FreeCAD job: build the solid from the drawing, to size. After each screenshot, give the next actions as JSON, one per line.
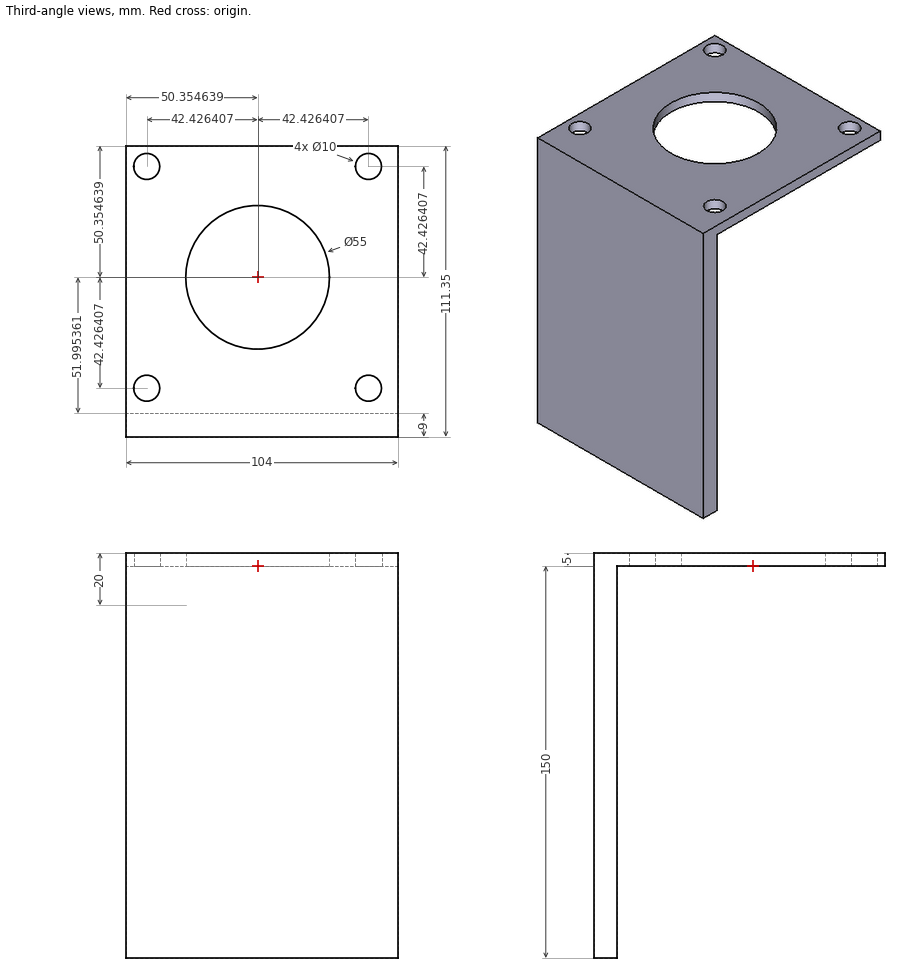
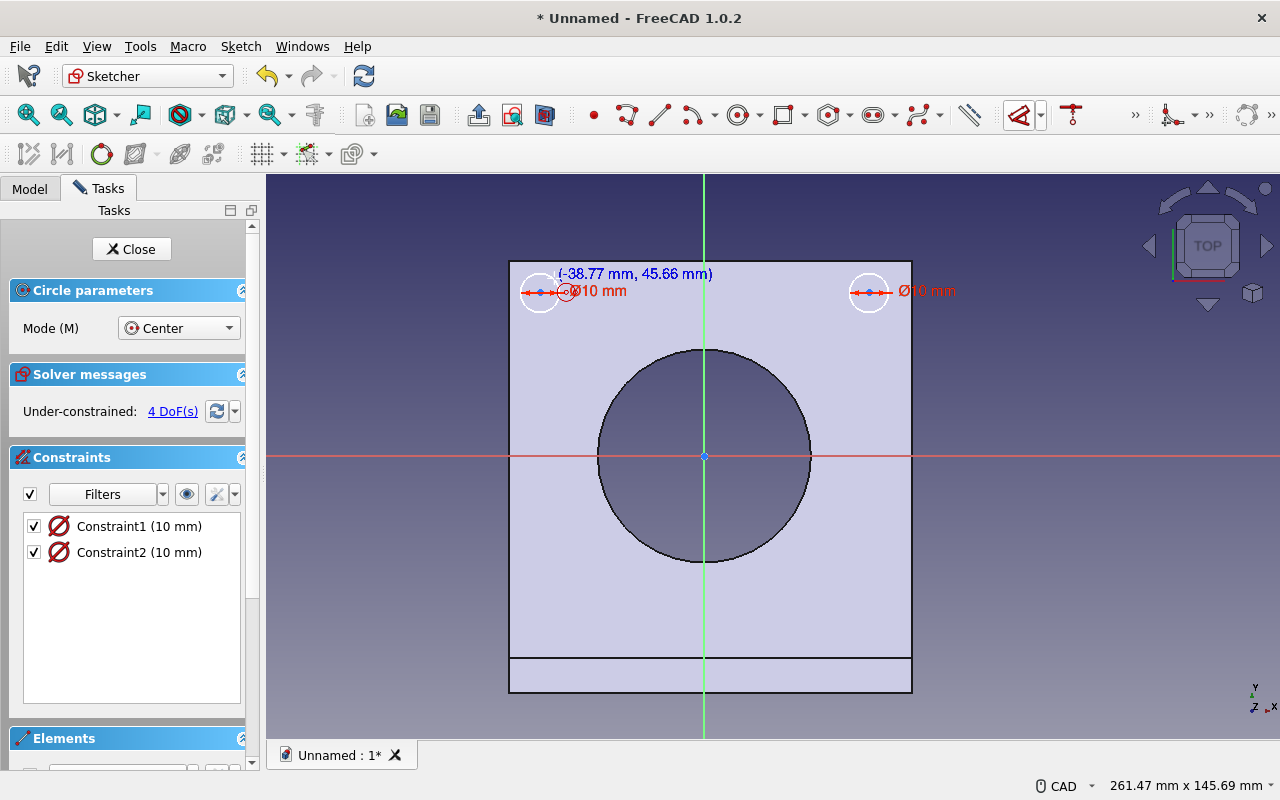
{"action": "left_click", "coordinate": [540, 621]}
{"action": "mouse_move", "coordinate": [554, 607]}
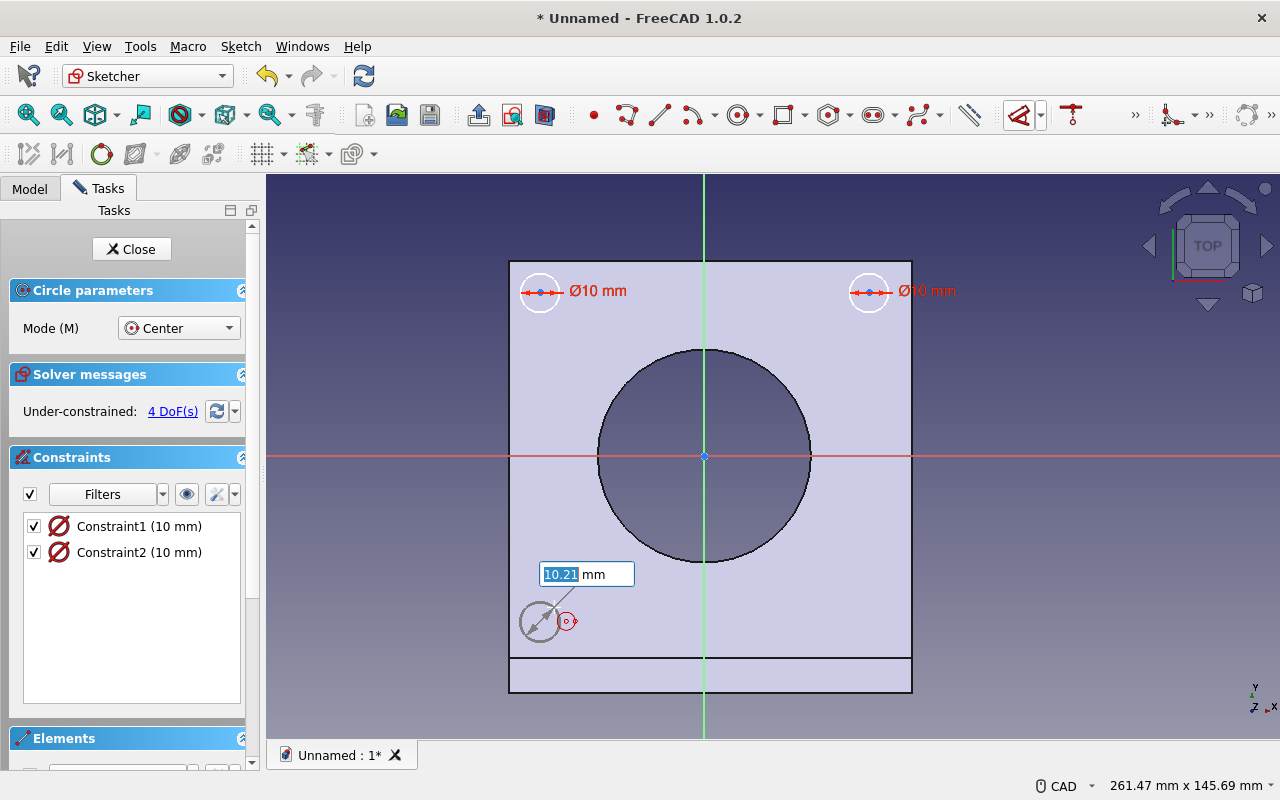
{"action": "type", "text": "10"}
{"action": "key", "text": "Return"}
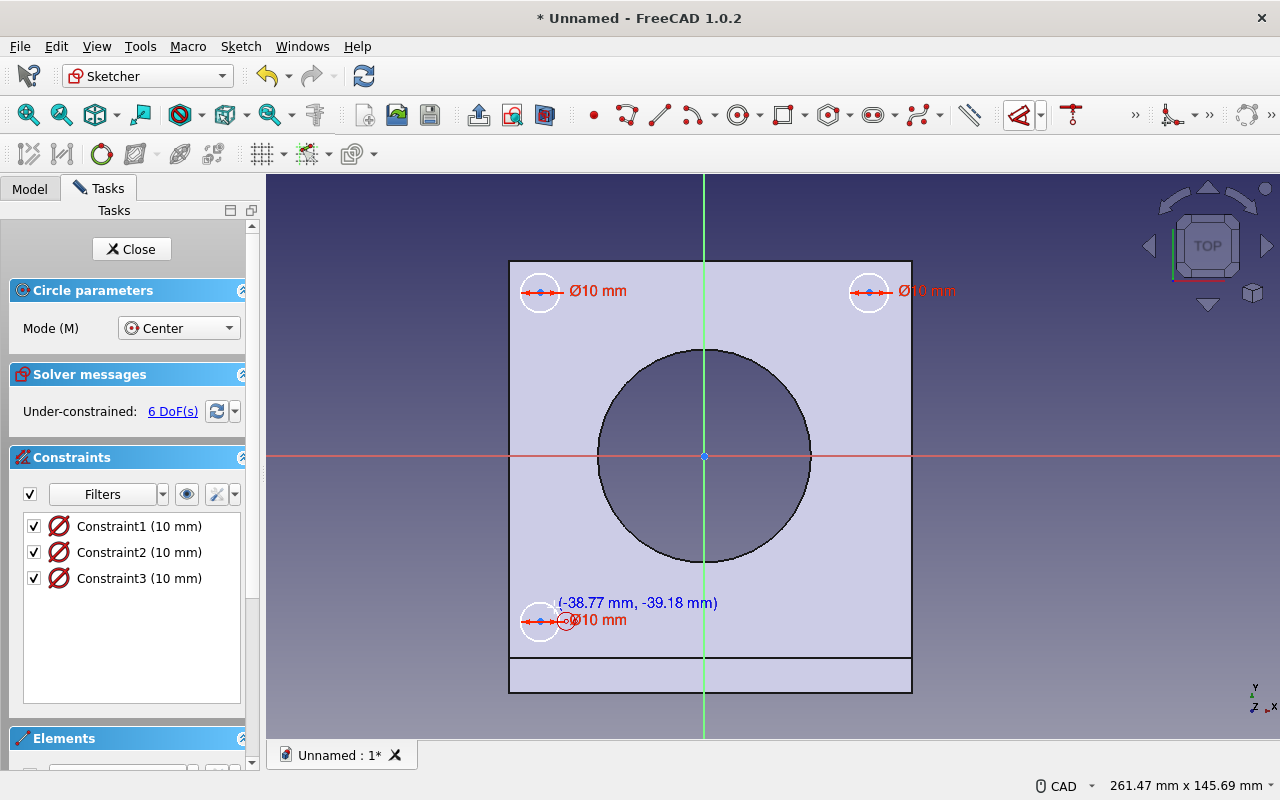
{"action": "left_click", "coordinate": [869, 621]}
{"action": "mouse_move", "coordinate": [883, 607]}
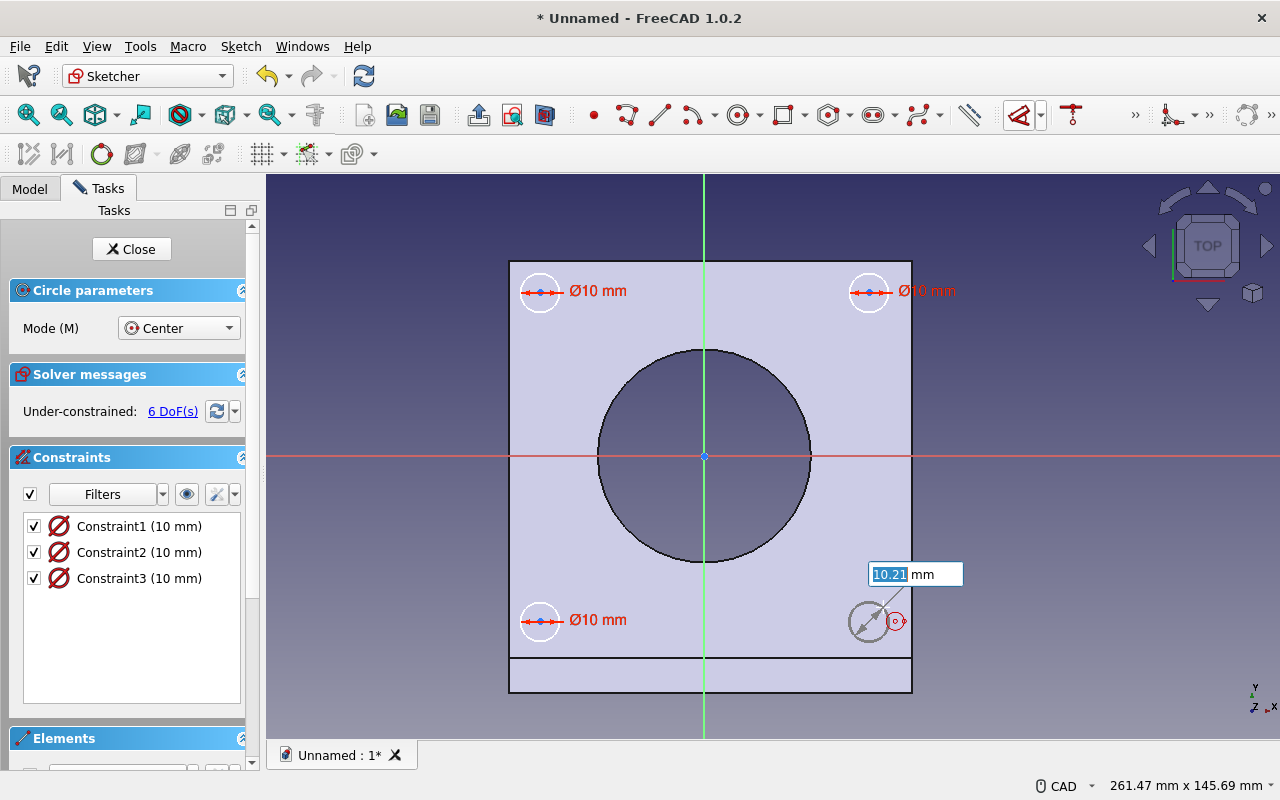
{"action": "type", "text": "10"}
{"action": "key", "text": "Return"}
{"action": "key", "text": "Escape"}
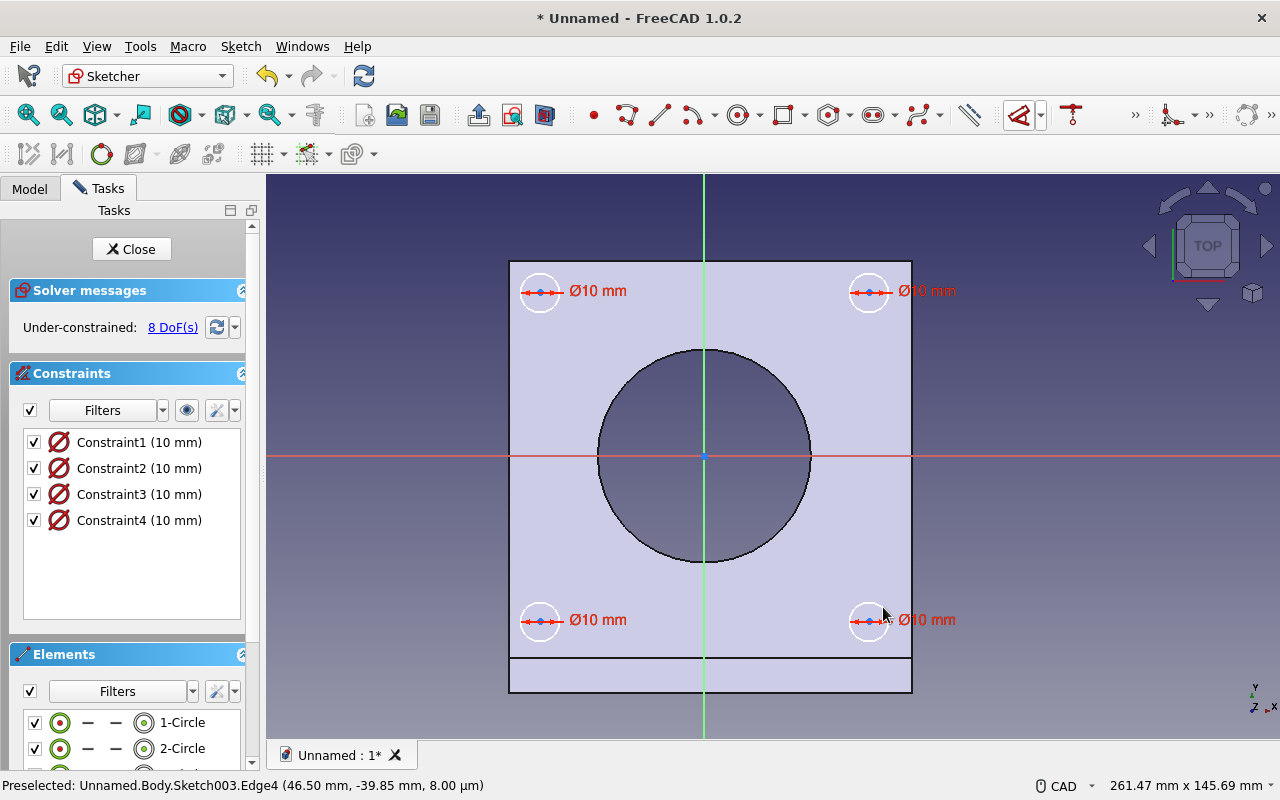
{"action": "left_click", "coordinate": [869, 293]}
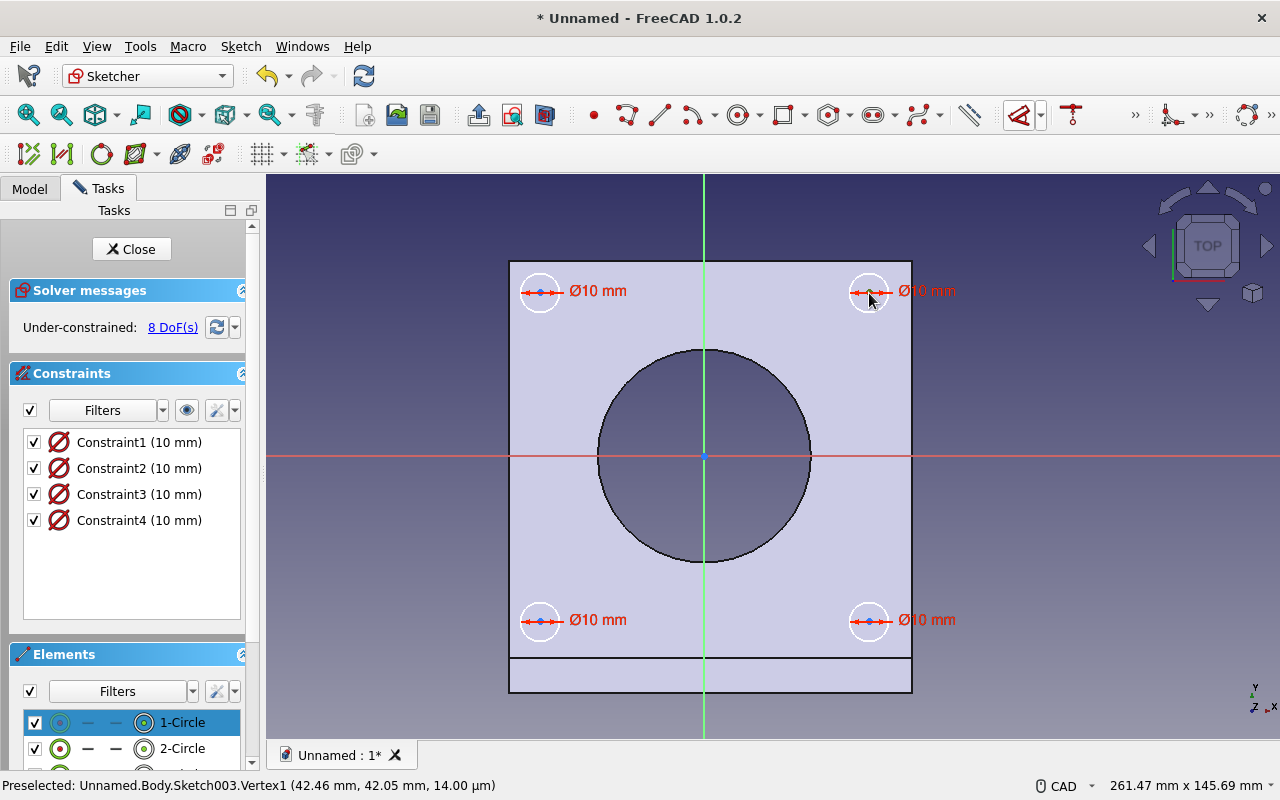
{"action": "left_click", "coordinate": [540, 293]}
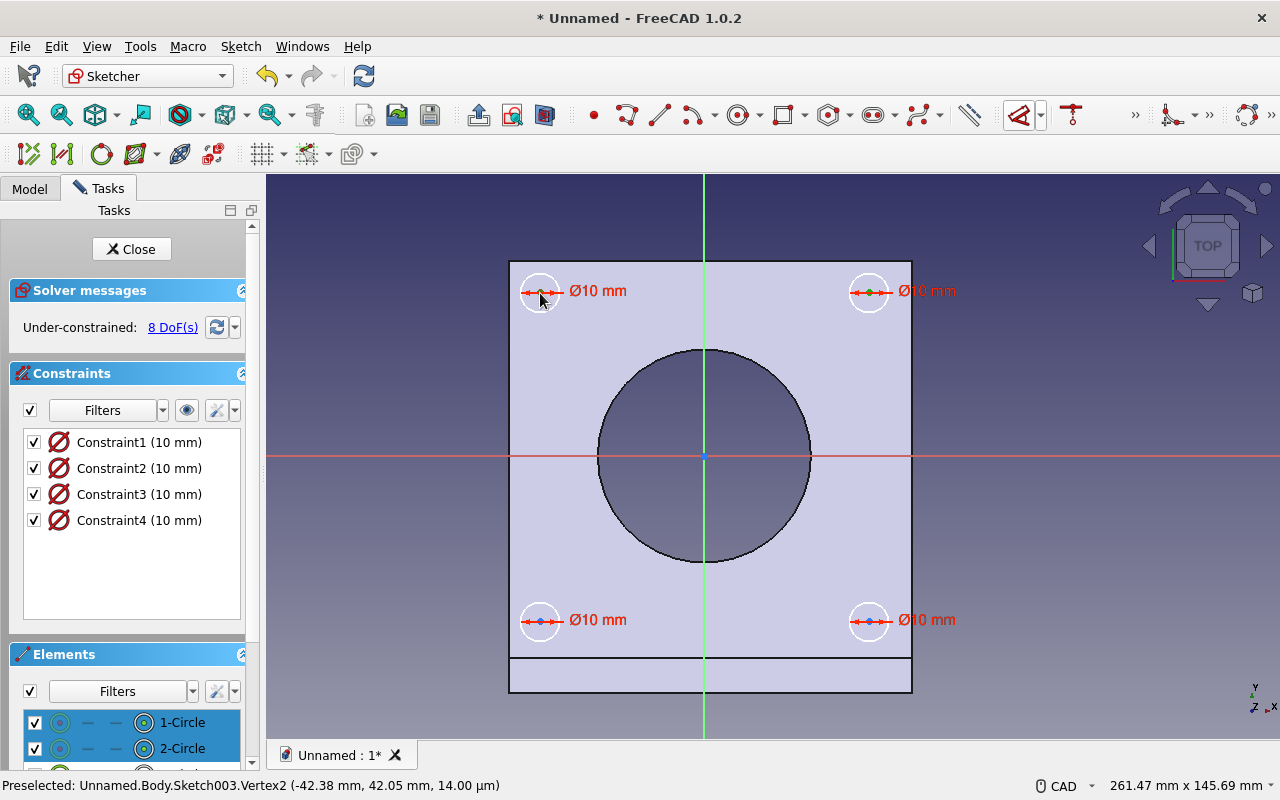
{"action": "key", "text": "h"}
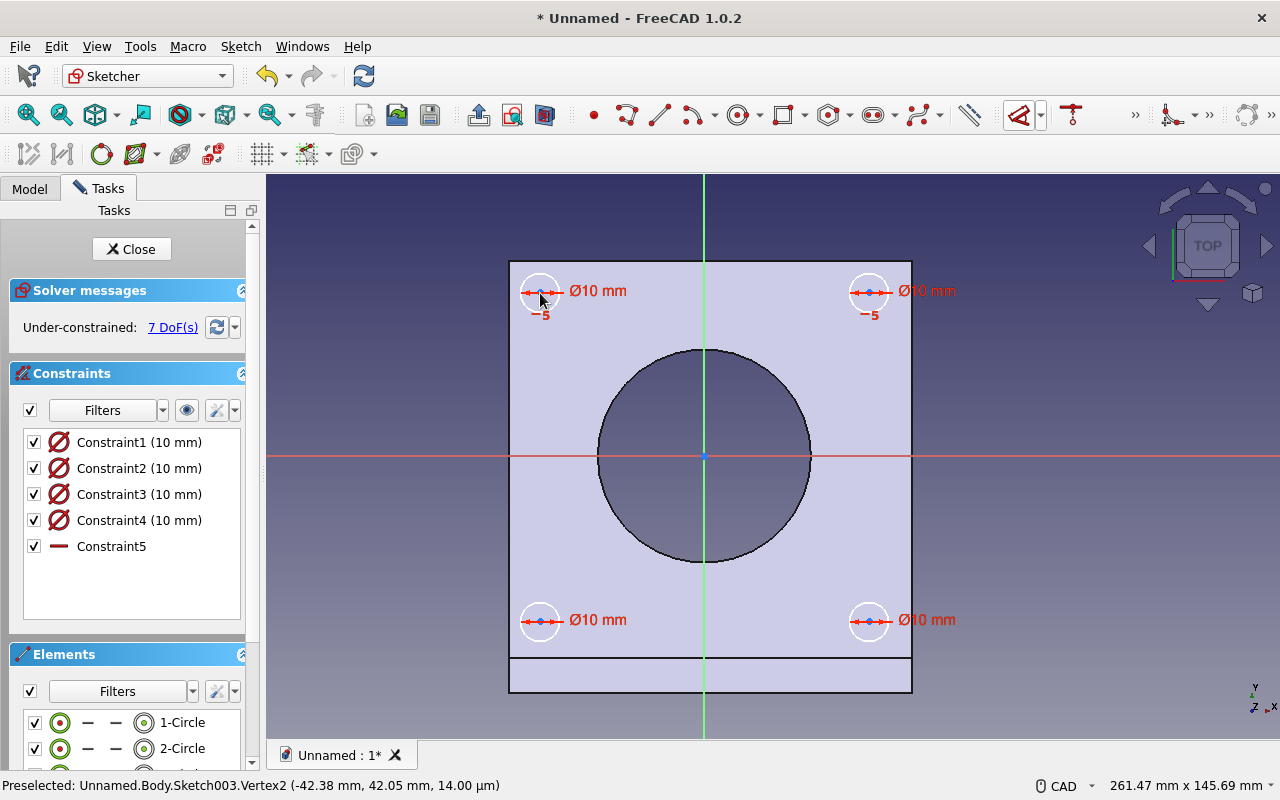
{"action": "left_click", "coordinate": [540, 293]}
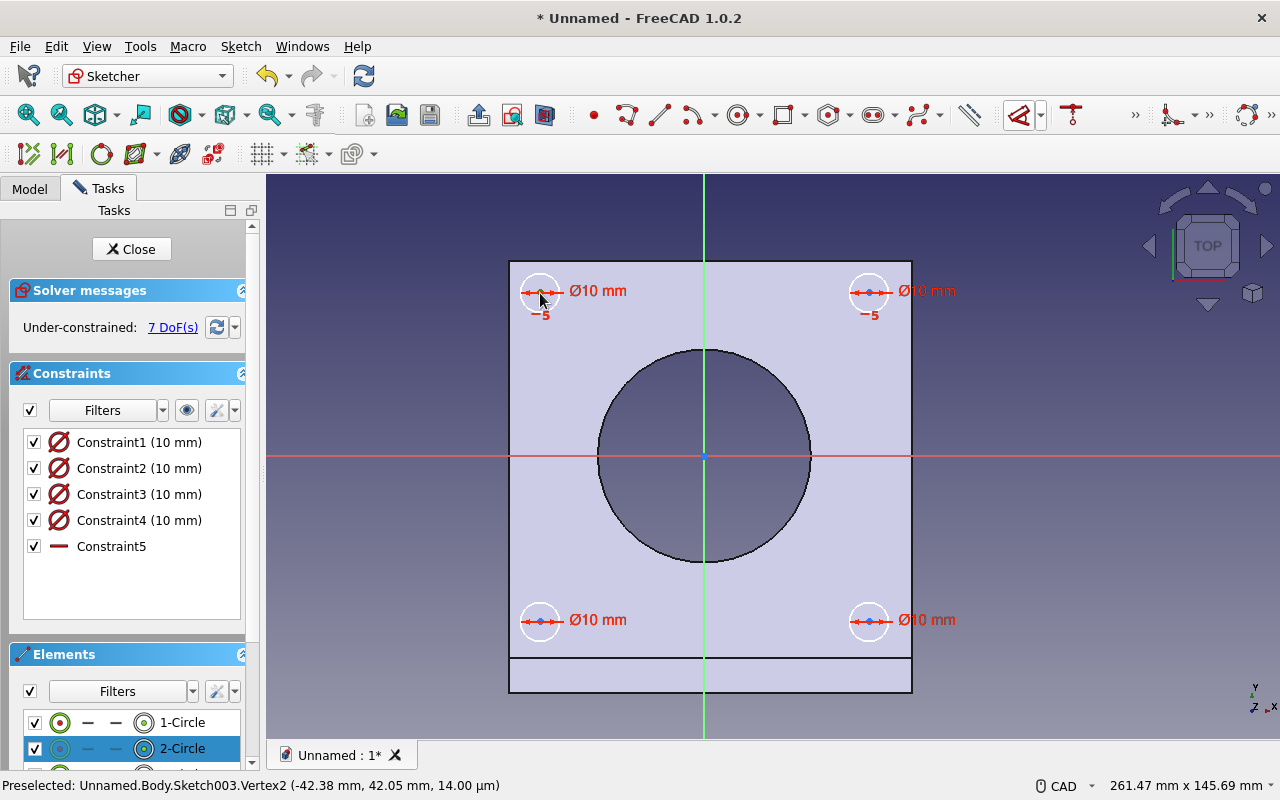
{"action": "left_click", "coordinate": [540, 622]}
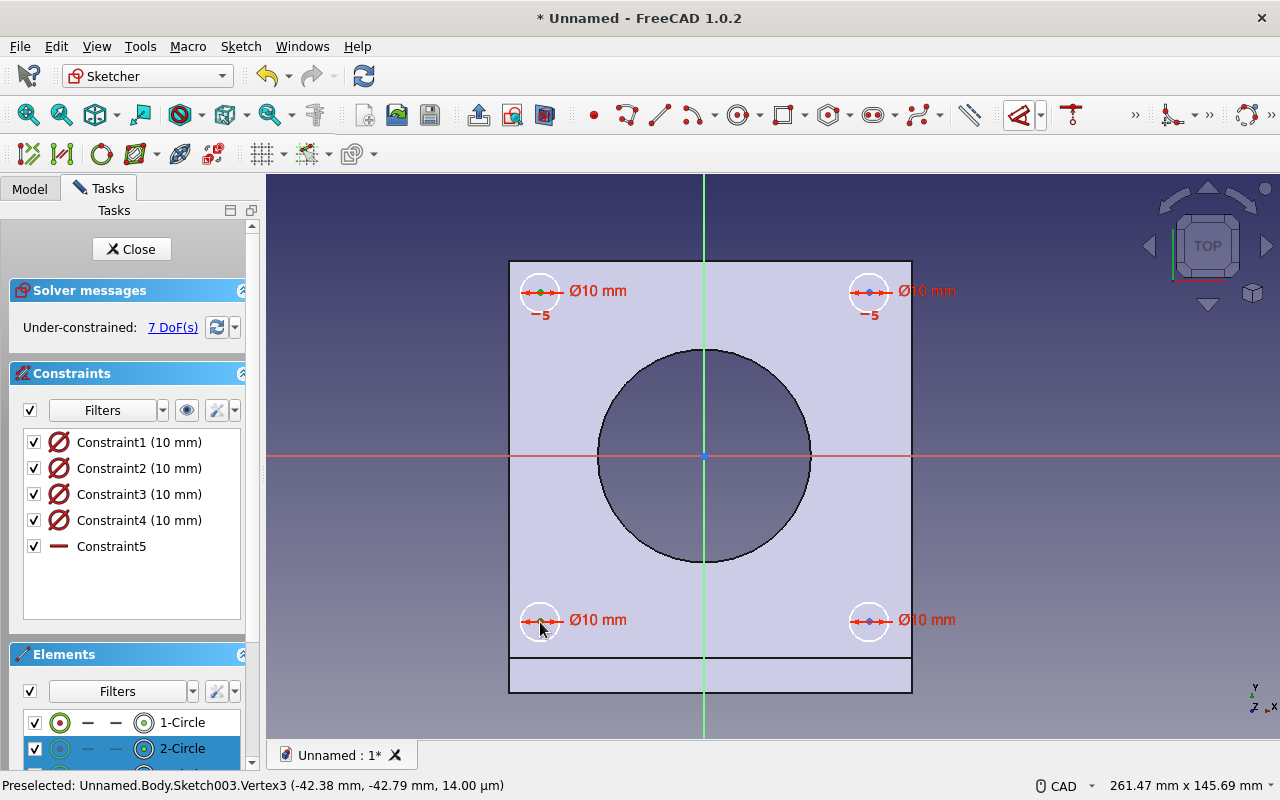
{"action": "key", "text": "v"}